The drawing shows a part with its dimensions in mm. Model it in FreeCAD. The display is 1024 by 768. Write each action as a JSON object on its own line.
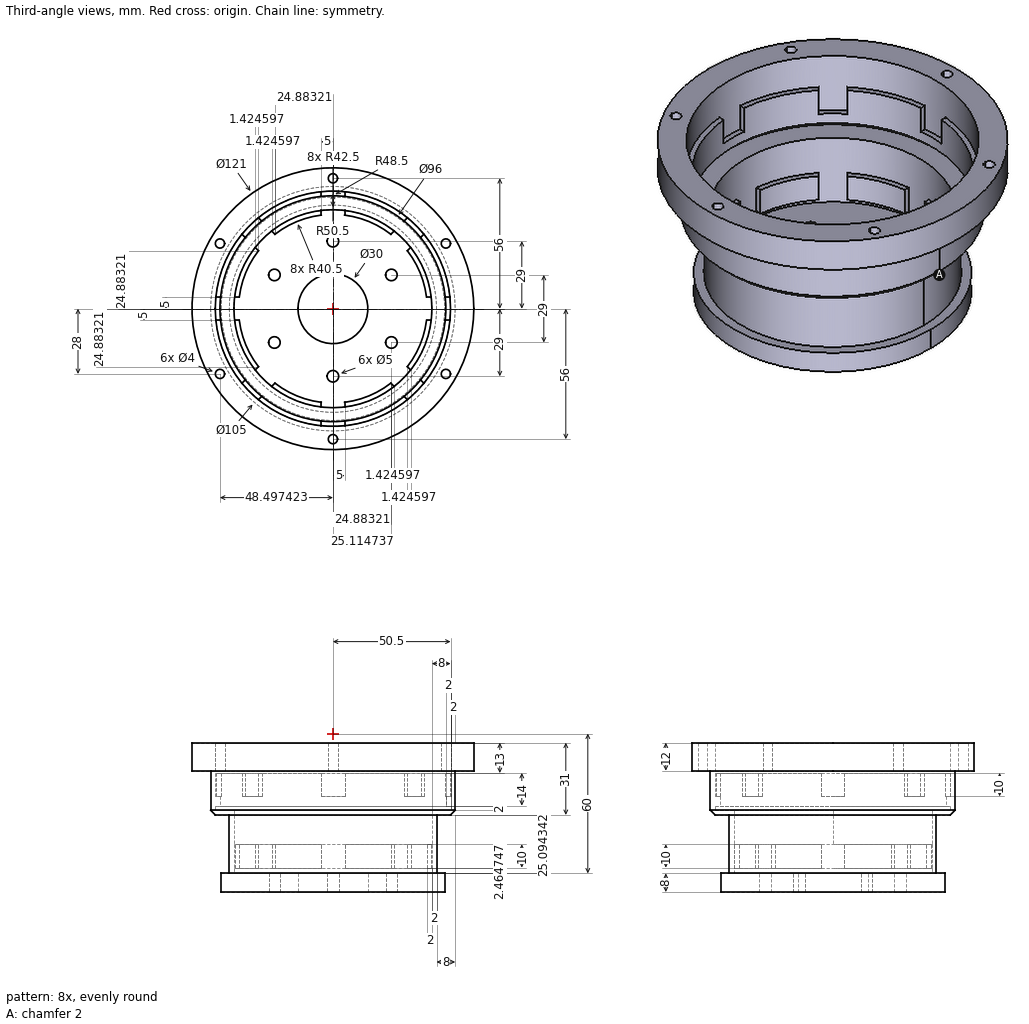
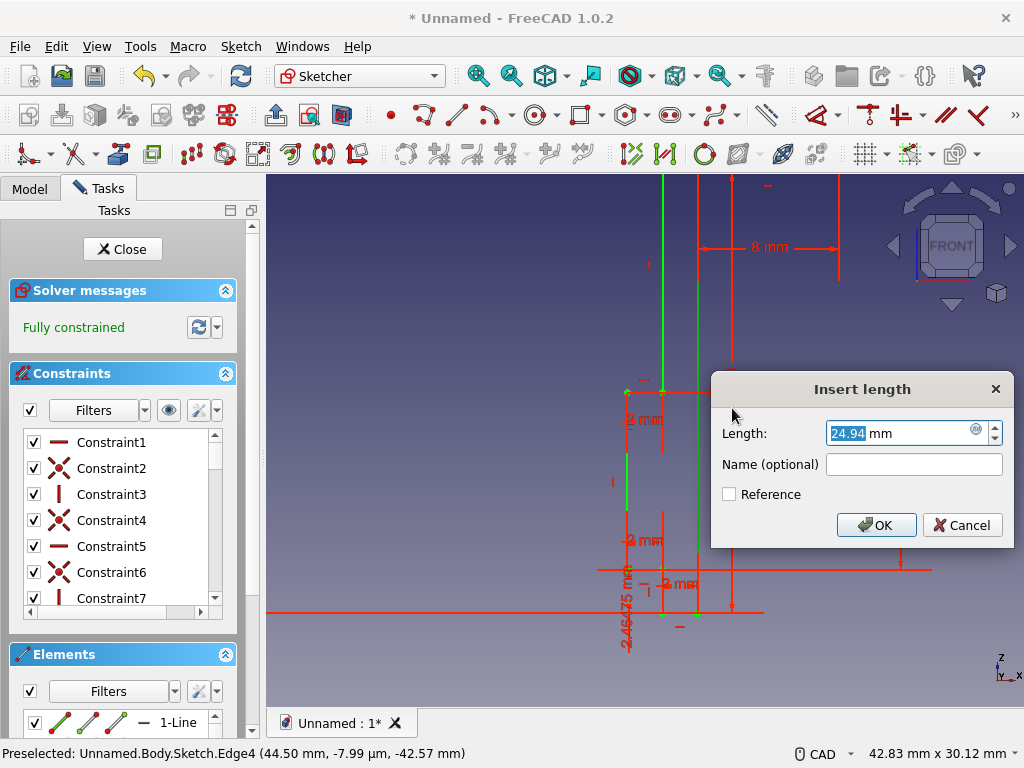
{"action": "type", "text": "25.094342"}
{"action": "key", "text": "Return"}
{"action": "key", "text": "Escape"}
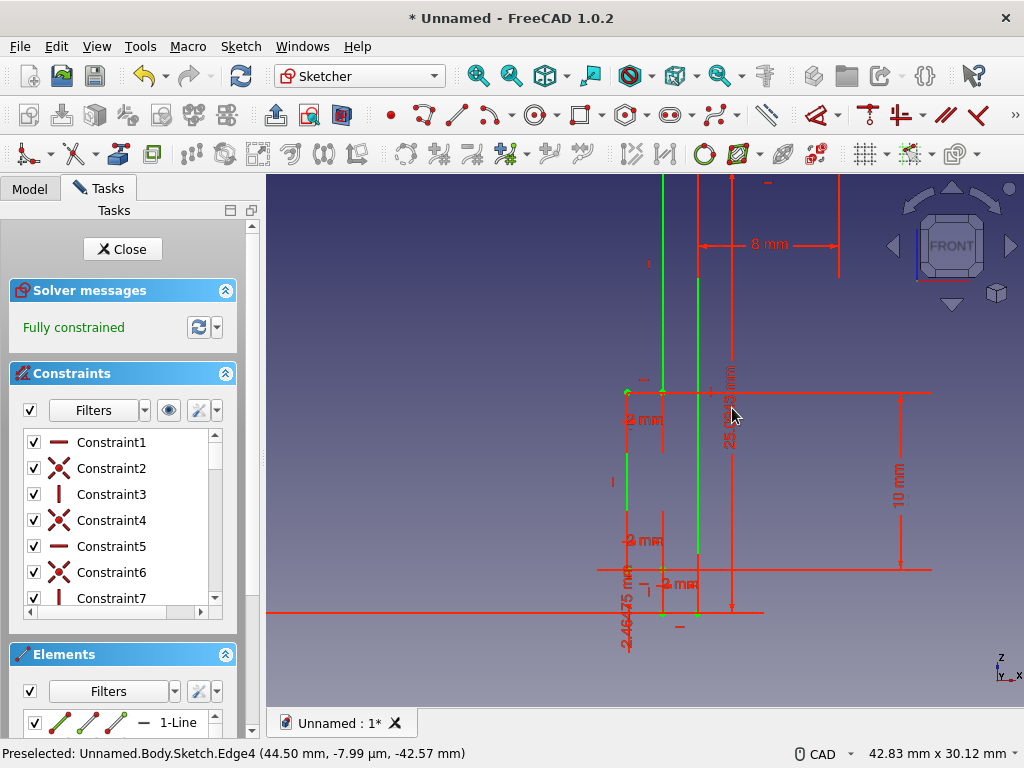
{"action": "left_click", "coordinate": [123, 249]}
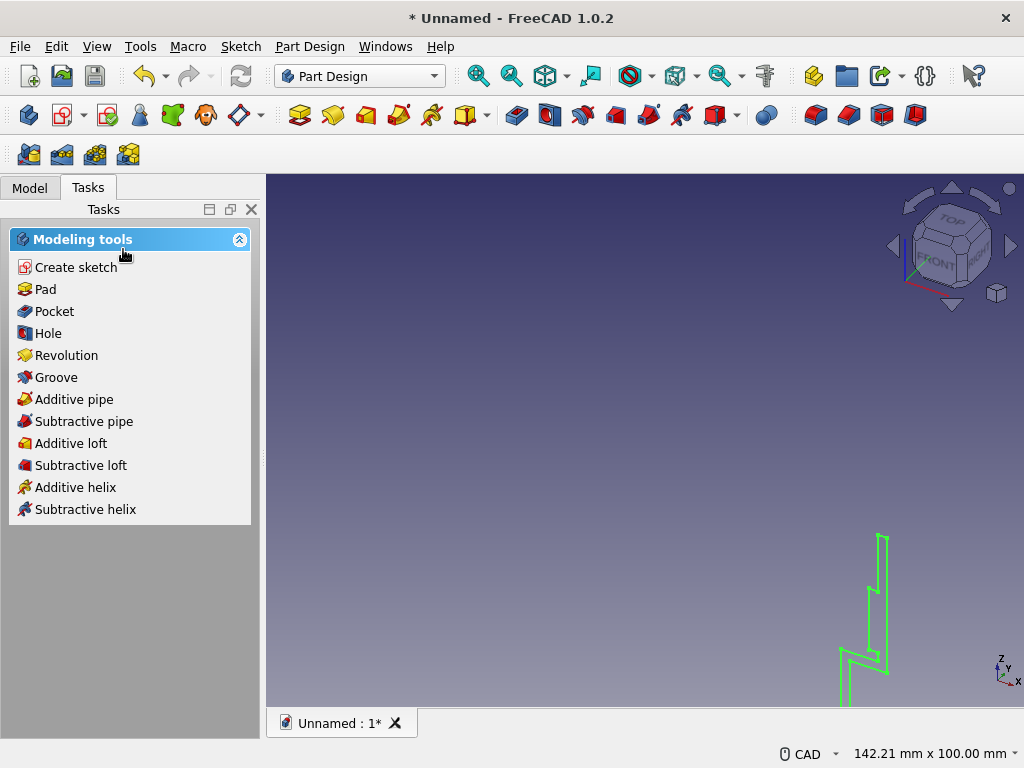
{"action": "left_click", "coordinate": [333, 116]}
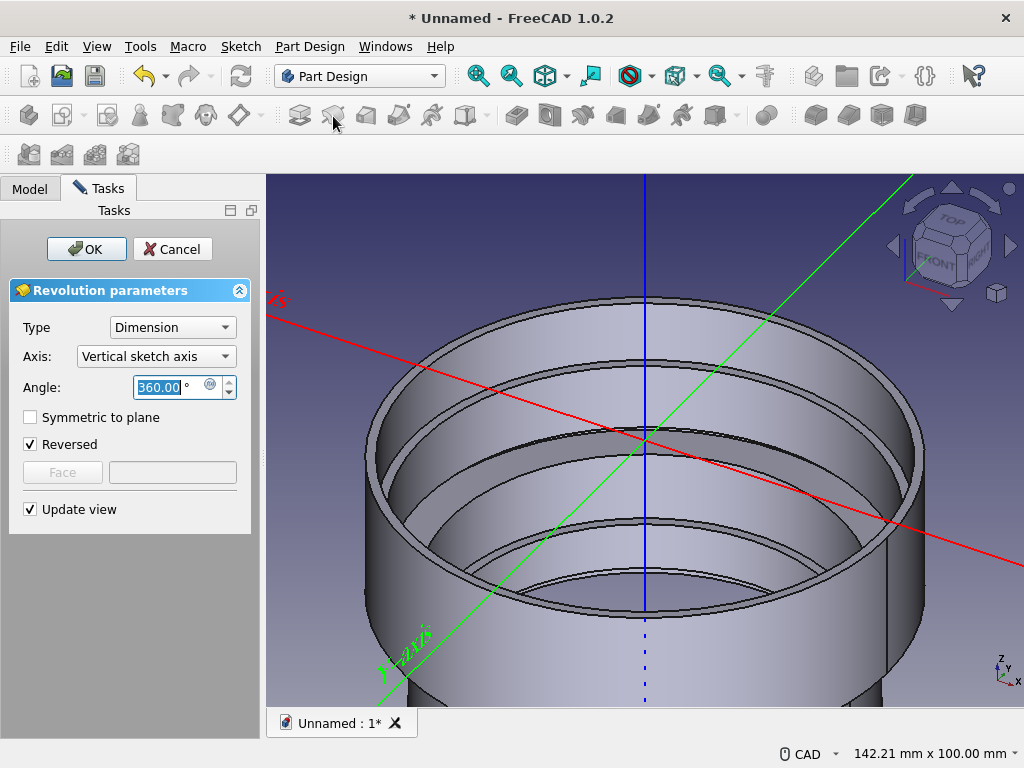
{"action": "left_click", "coordinate": [87, 249]}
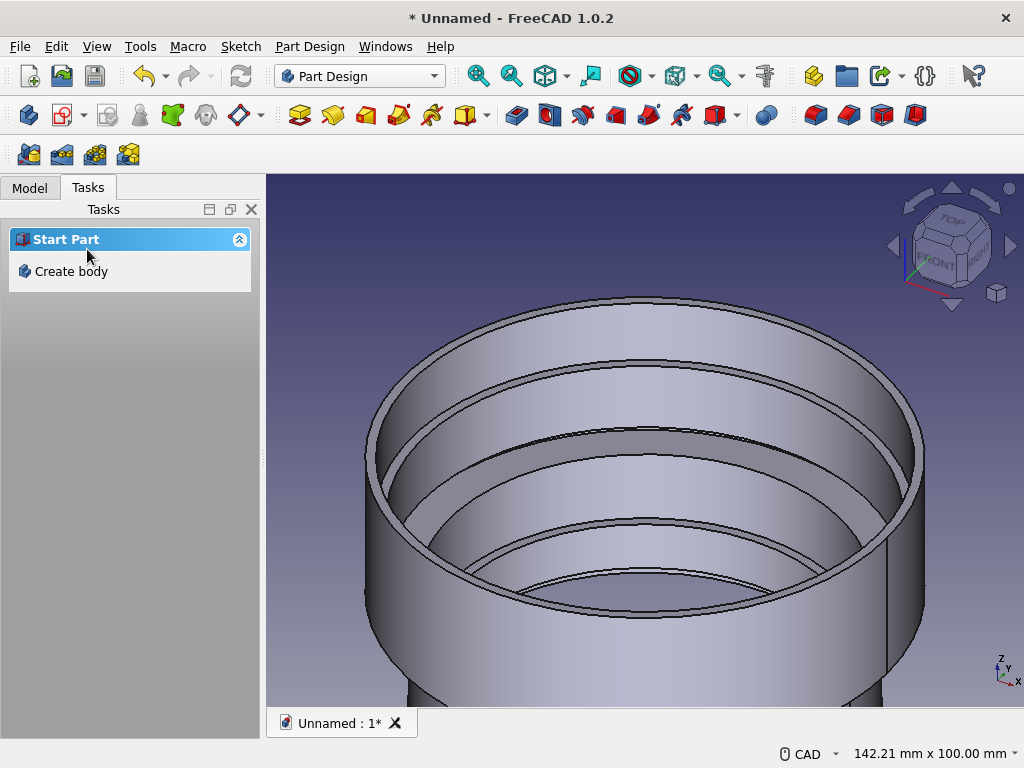
{"action": "key", "text": "v f"}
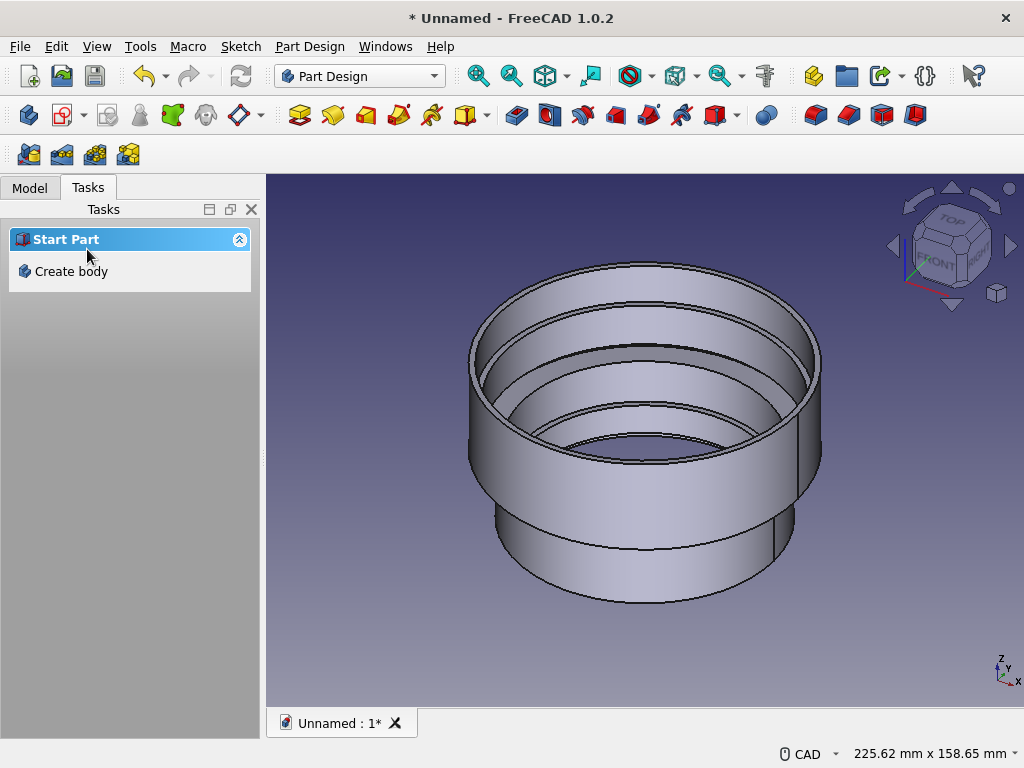
{"action": "key", "text": "5"}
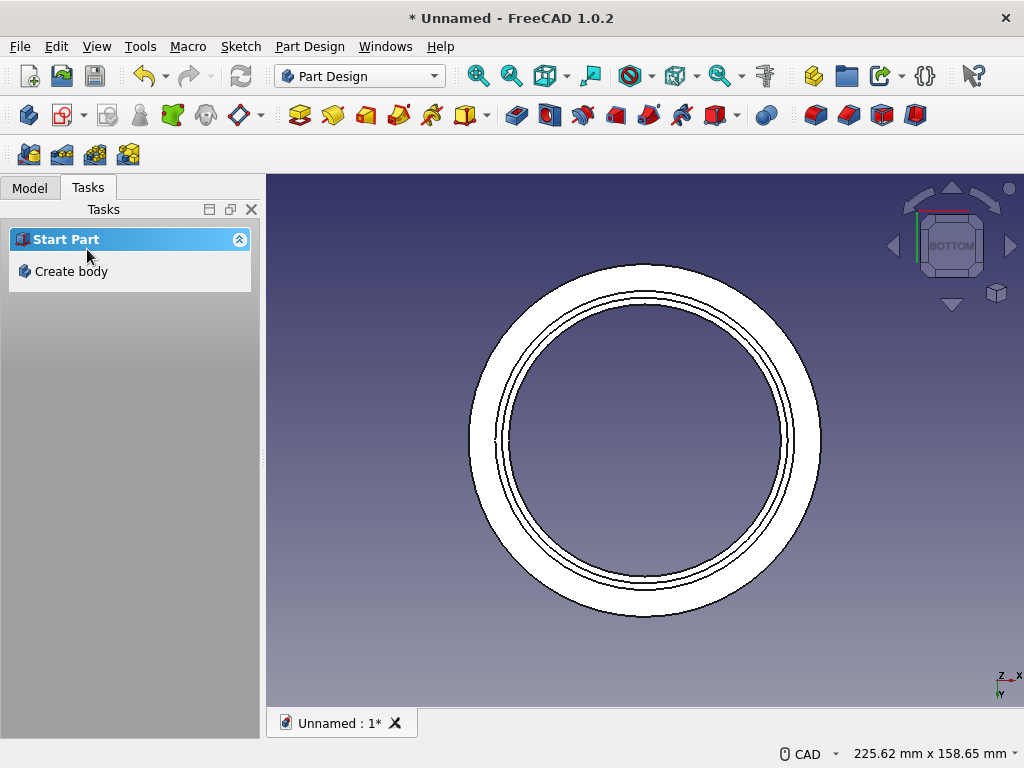
{"action": "scroll", "coordinate": [573, 560], "scroll_direction": "up", "scroll_amount": 9}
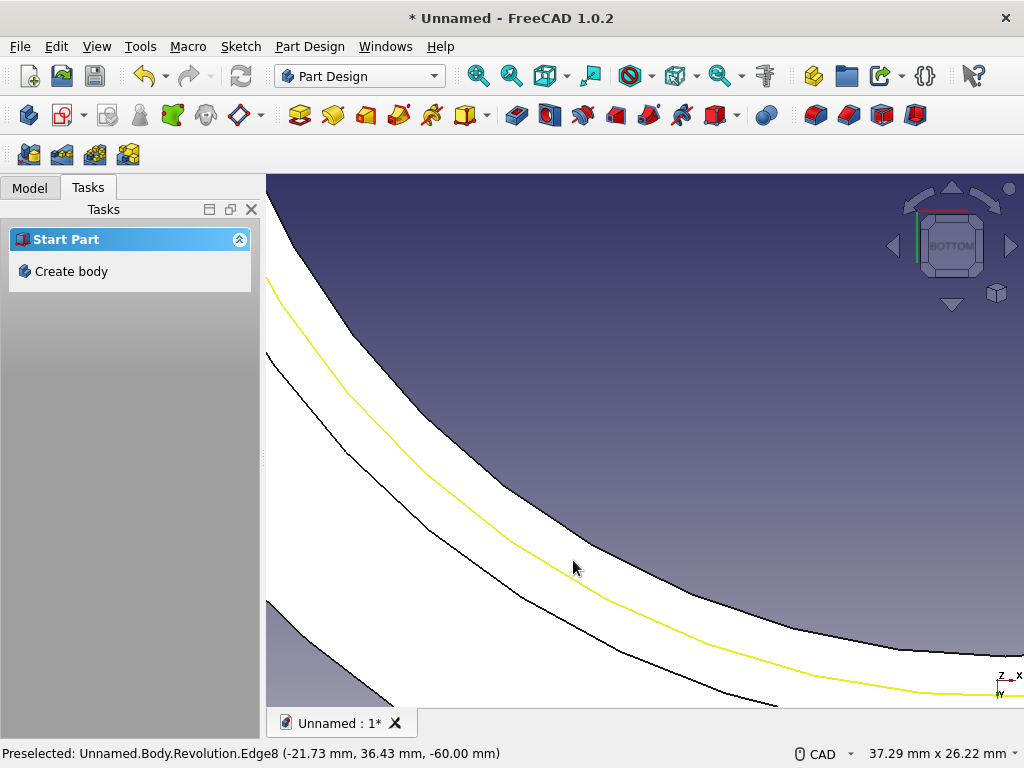
{"action": "left_click", "coordinate": [568, 561]}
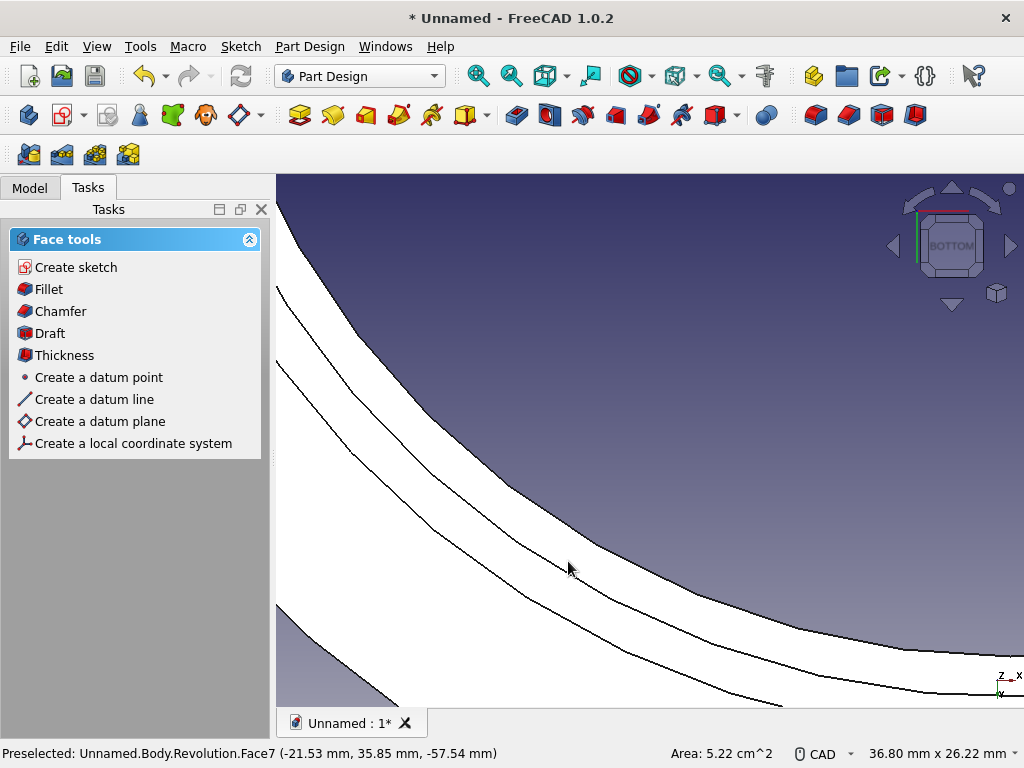
{"action": "left_click", "coordinate": [62, 116]}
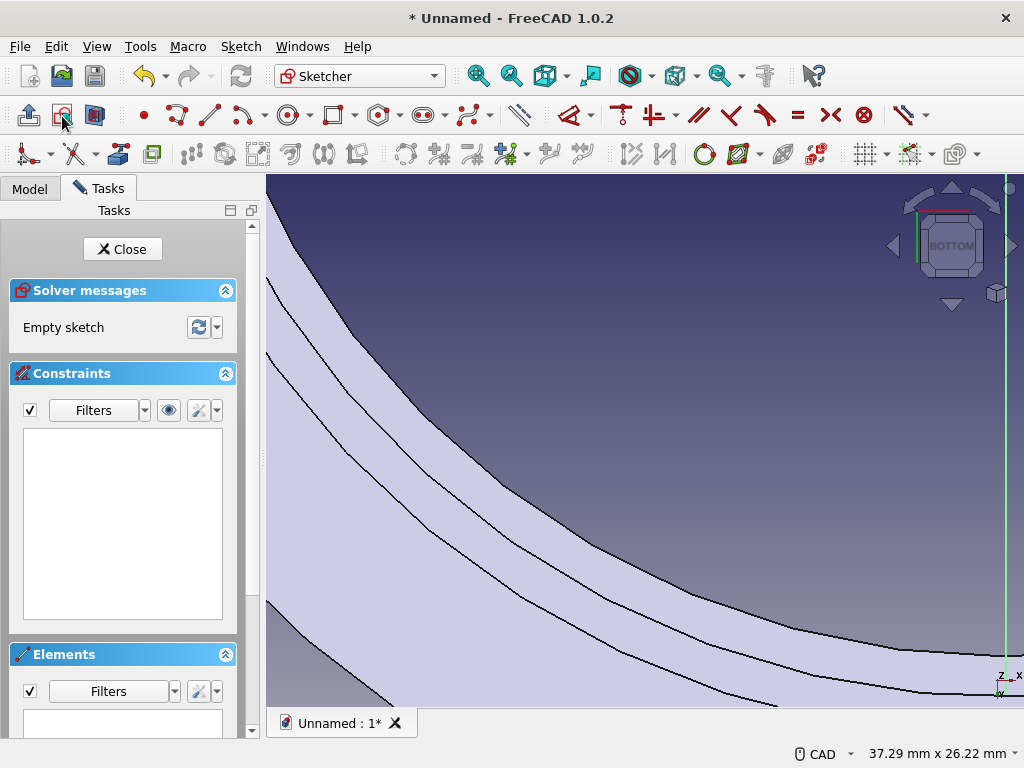
{"action": "scroll", "coordinate": [468, 594], "scroll_direction": "down", "scroll_amount": 8}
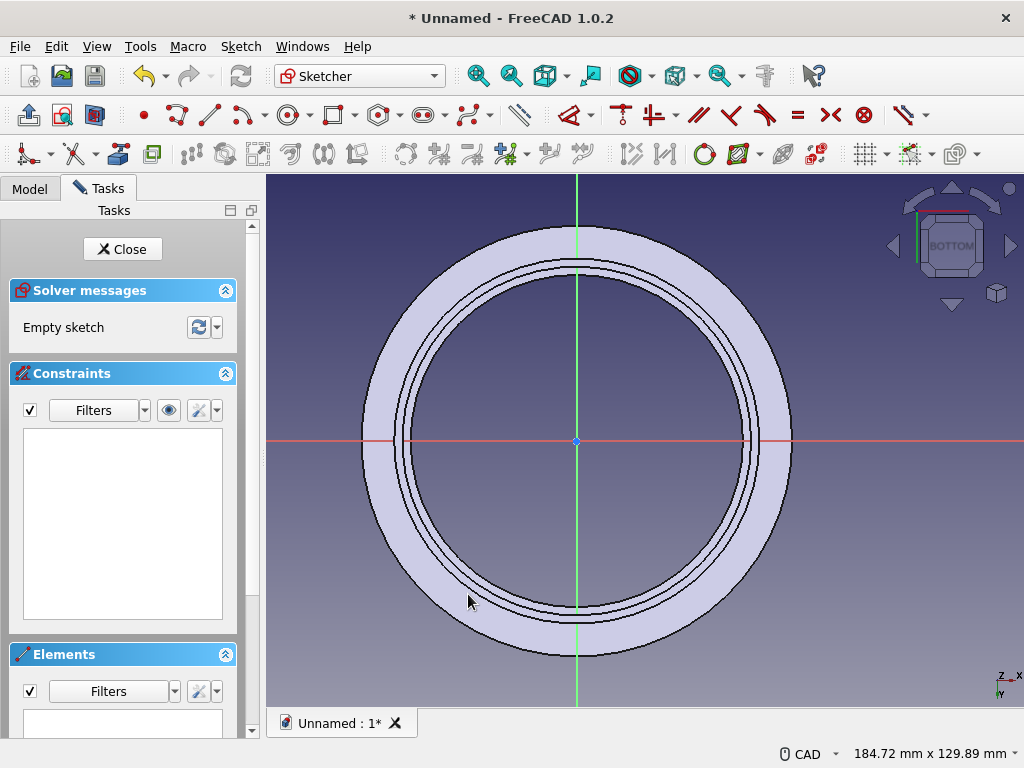
{"action": "key", "text": "g l"}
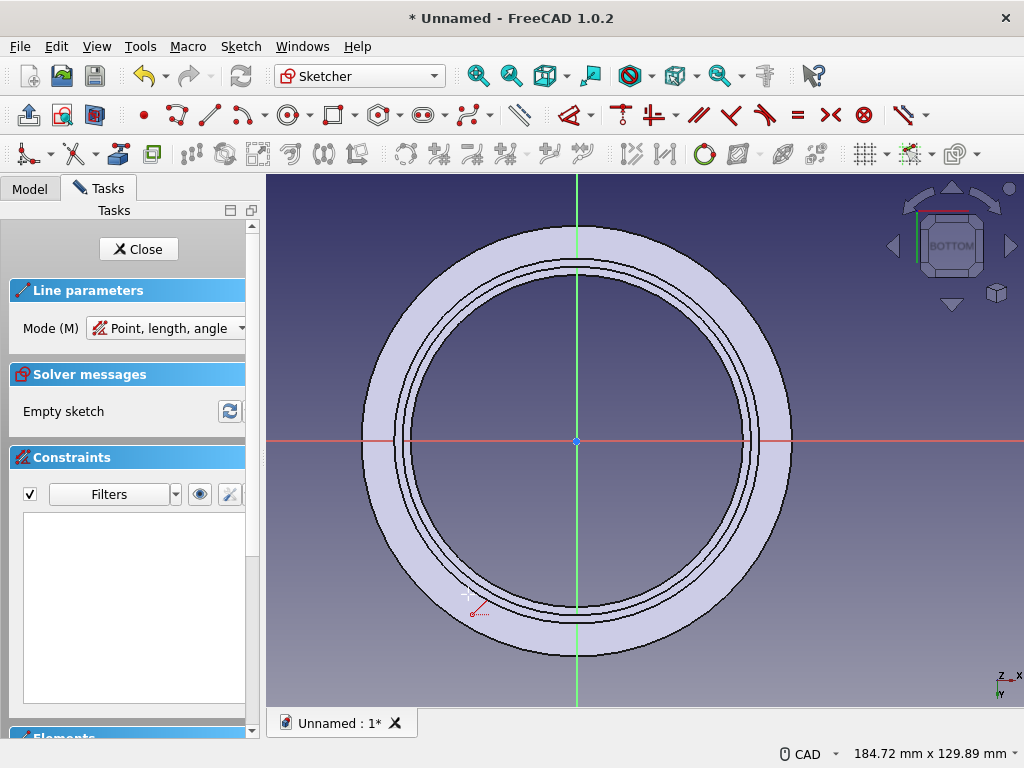
{"action": "left_click", "coordinate": [556, 614]}